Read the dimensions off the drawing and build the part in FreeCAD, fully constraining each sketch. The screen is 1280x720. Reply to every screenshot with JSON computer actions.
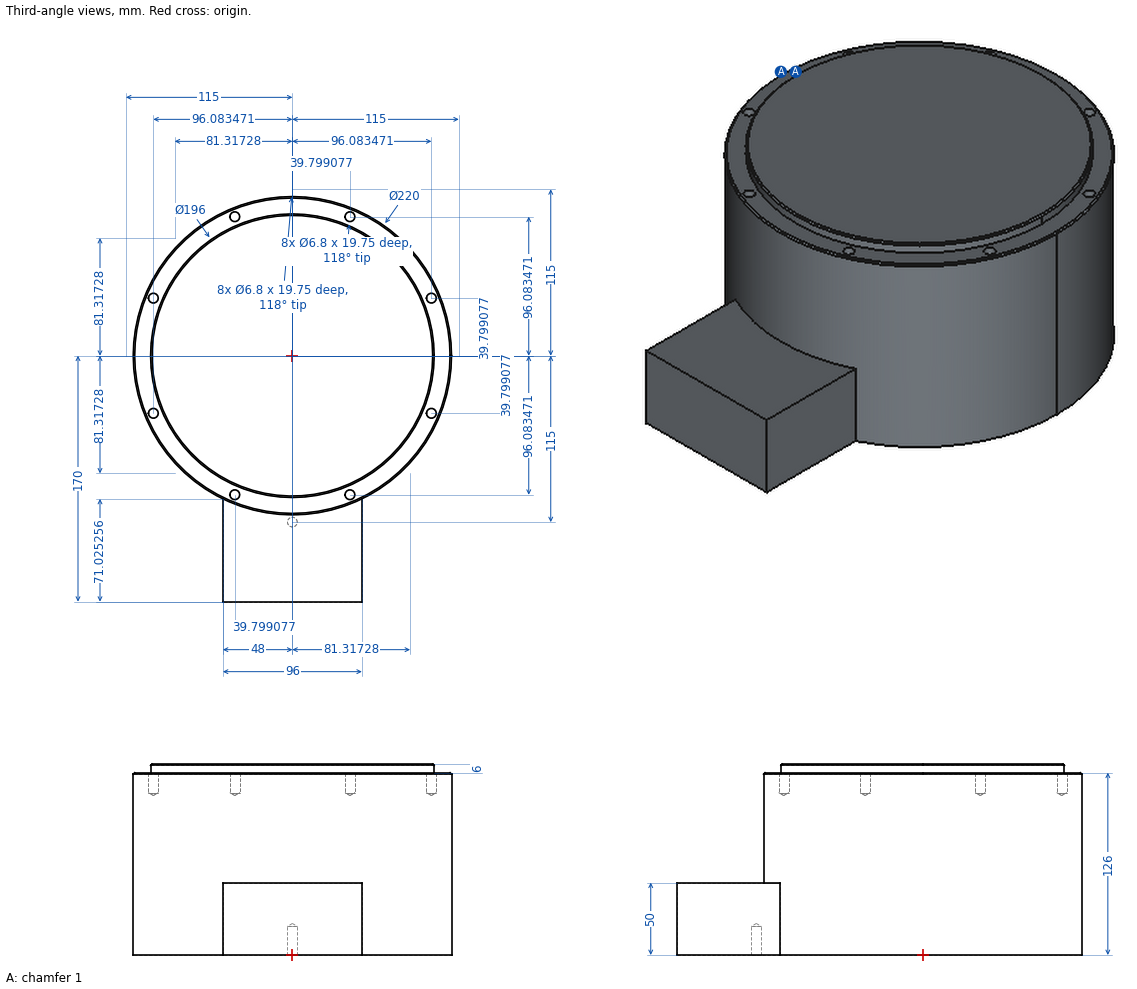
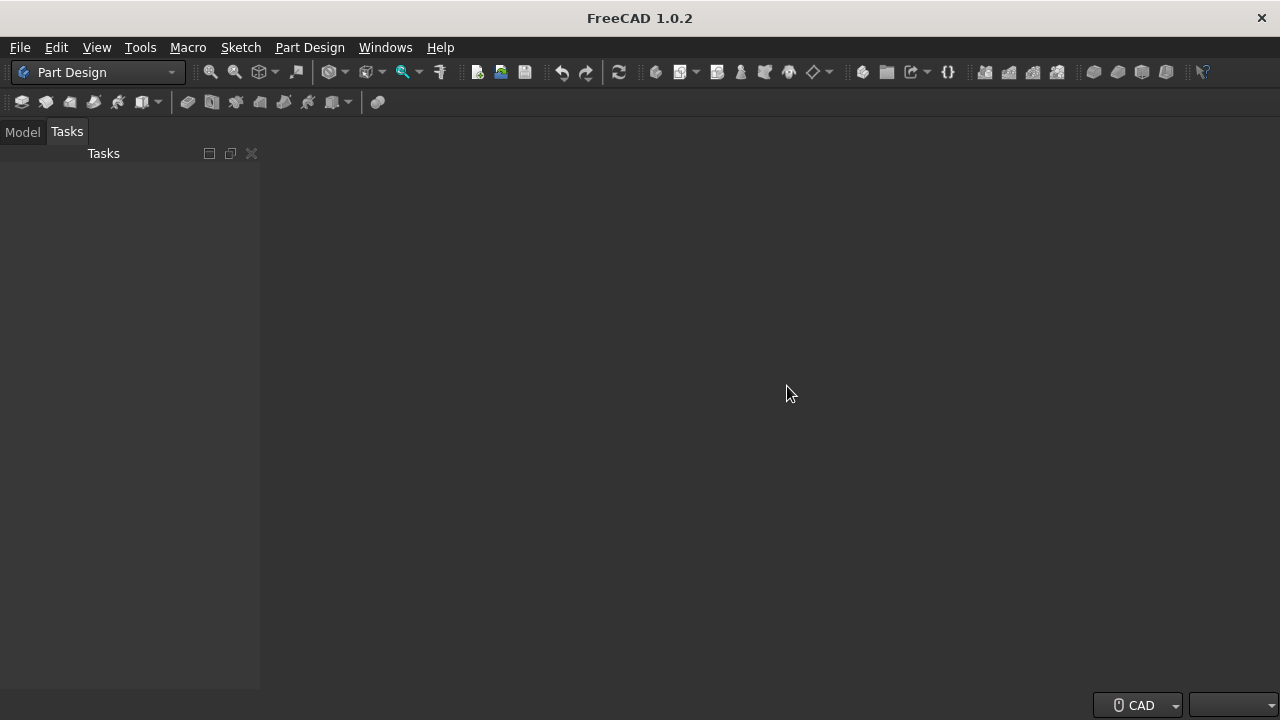
{"action": "left_click", "coordinate": [478, 72]}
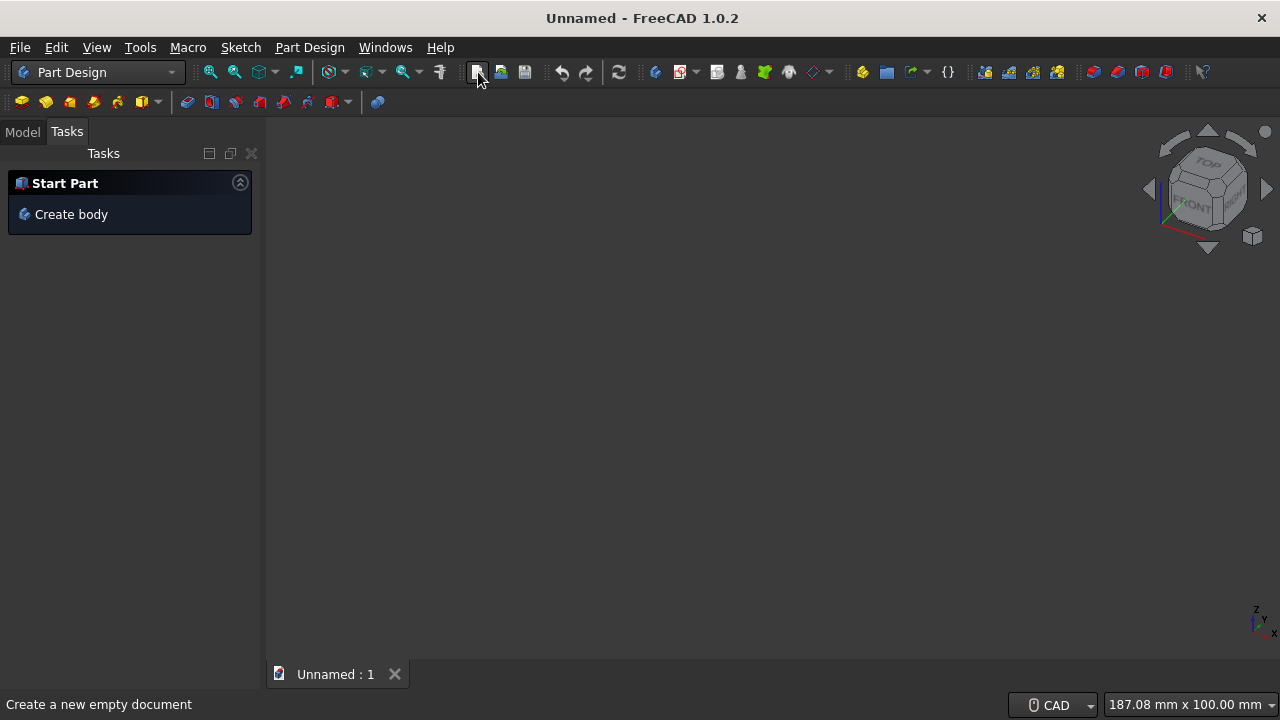
{"action": "left_click", "coordinate": [680, 72]}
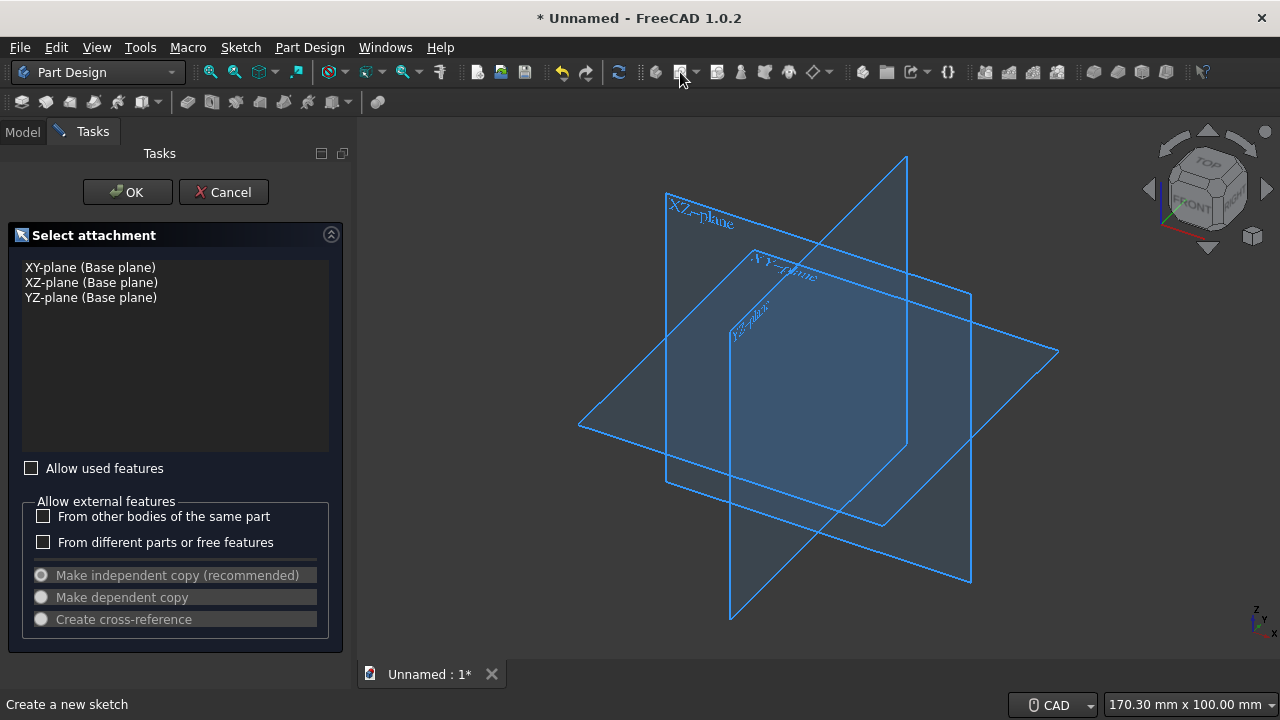
{"action": "left_click", "coordinate": [82, 268]}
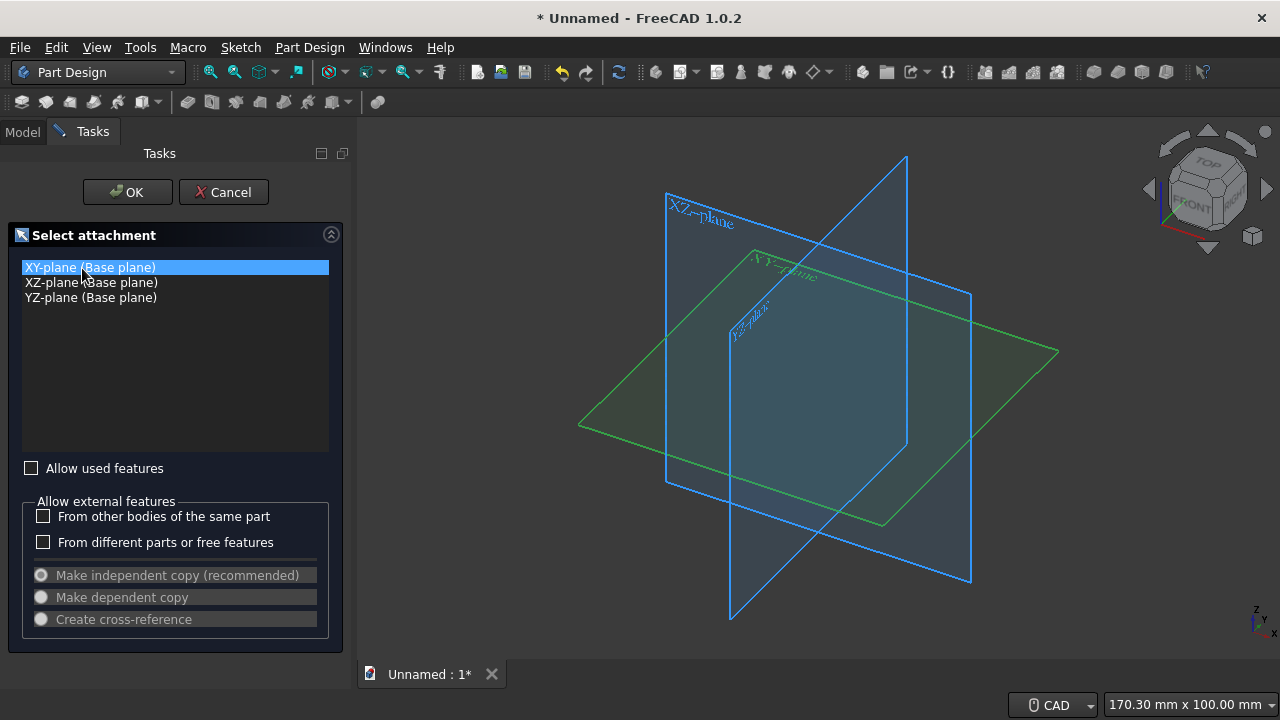
{"action": "left_click", "coordinate": [128, 192]}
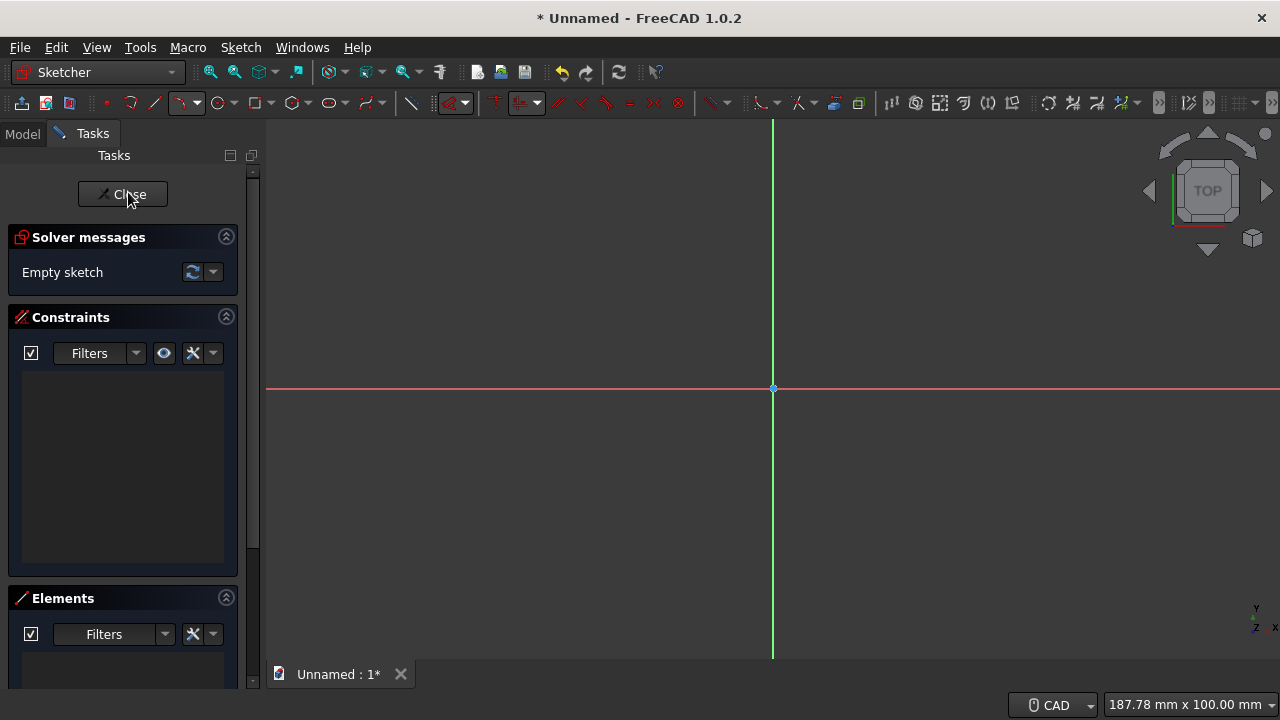
{"action": "scroll", "coordinate": [675, 389], "scroll_direction": "down", "scroll_amount": 6}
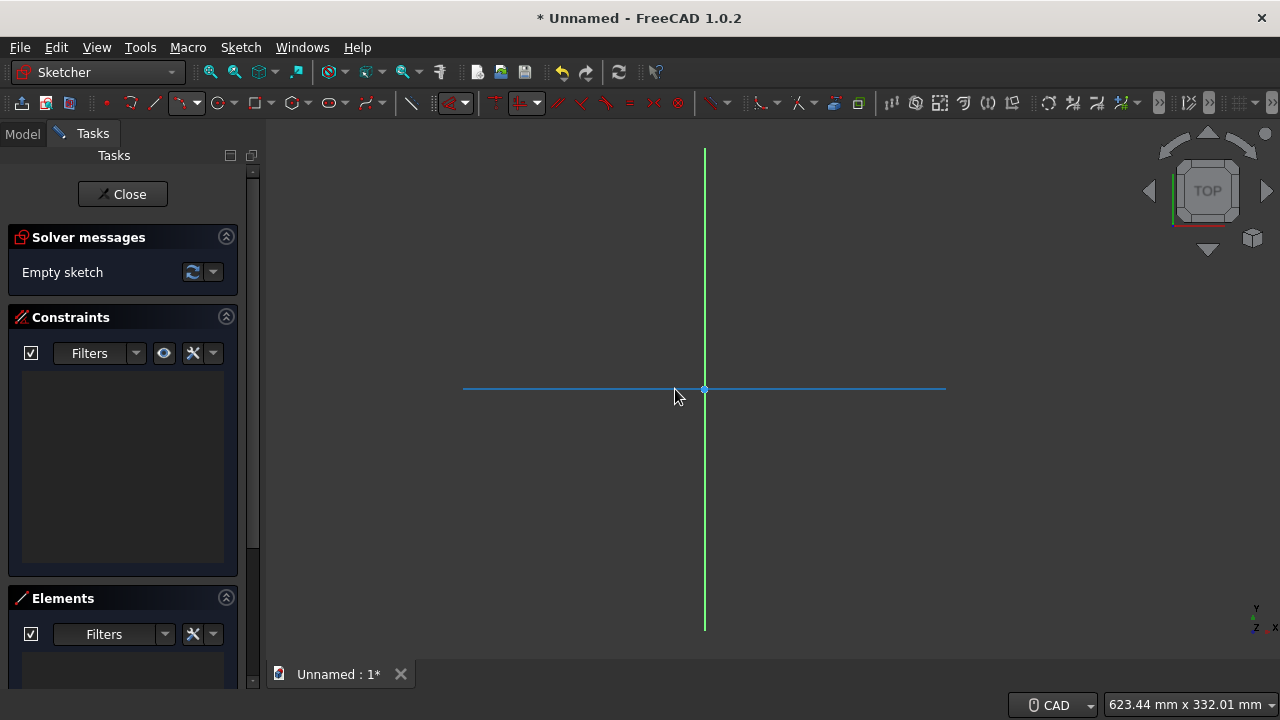
{"action": "left_click", "coordinate": [218, 104]}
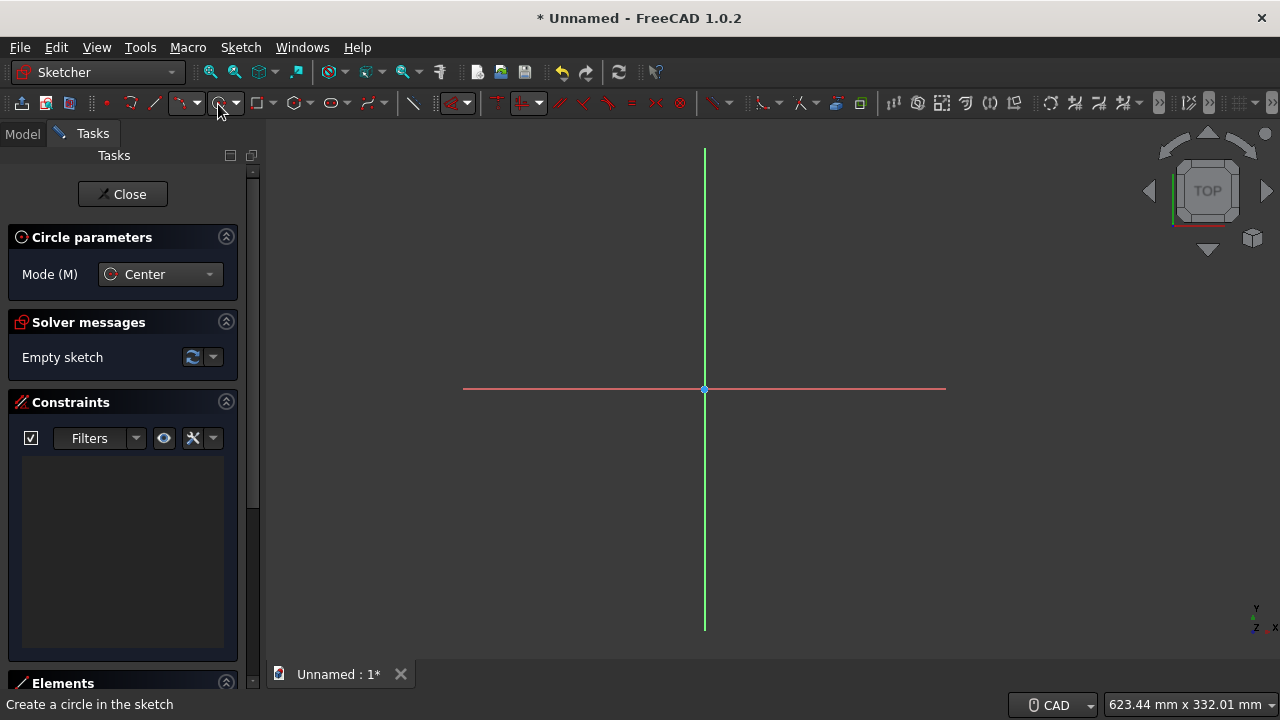
{"action": "left_click", "coordinate": [705, 389]}
{"action": "left_click", "coordinate": [831, 263]}
{"action": "key", "text": "Escape"}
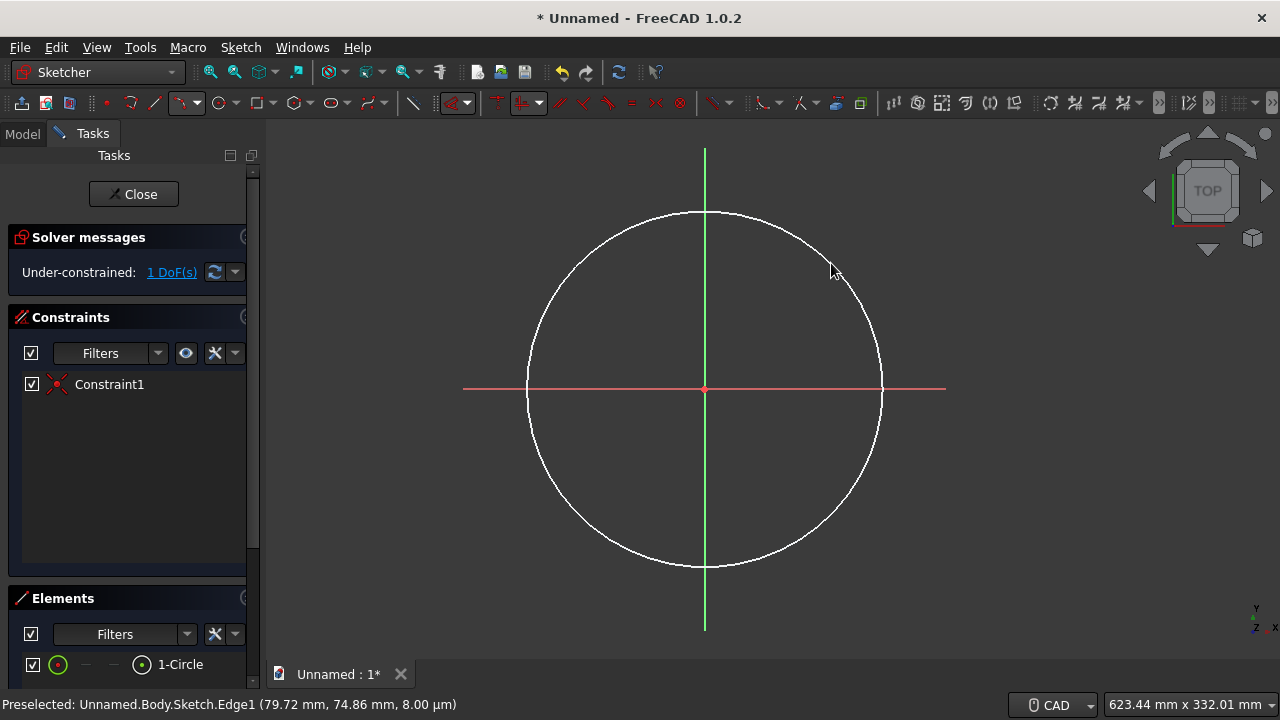
{"action": "left_click", "coordinate": [452, 104]}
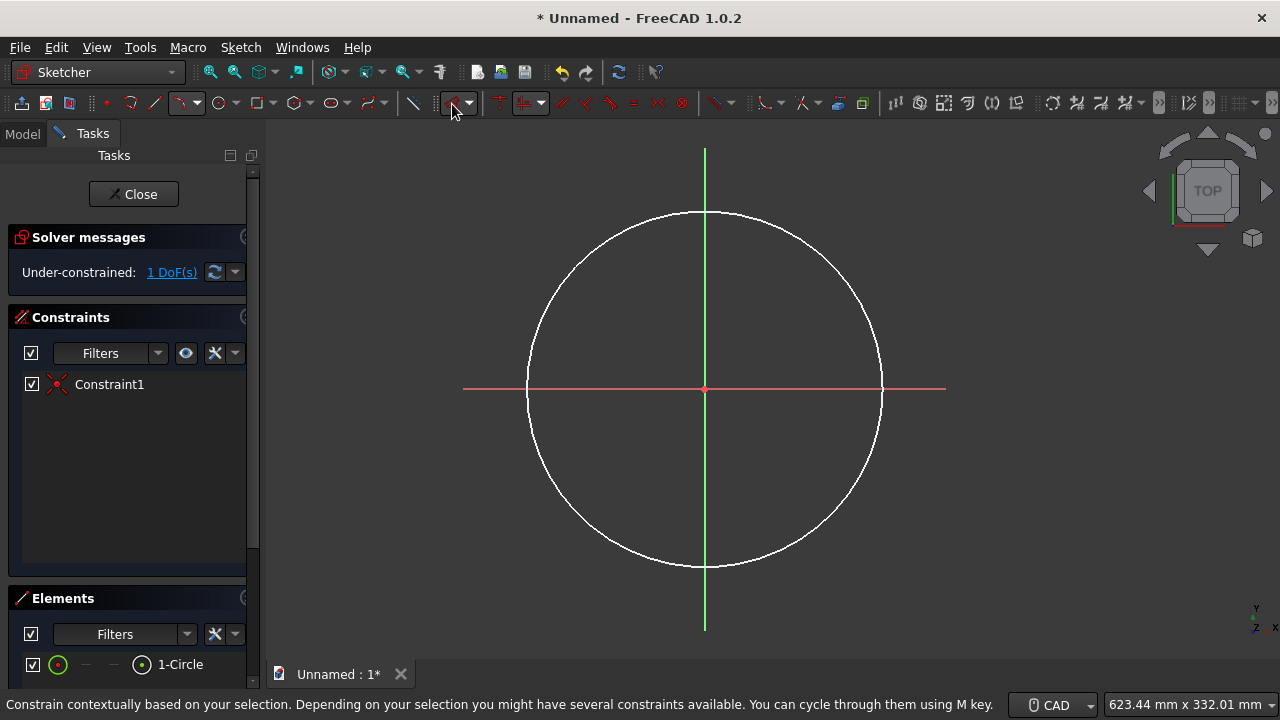
{"action": "left_click", "coordinate": [830, 263]}
{"action": "left_click", "coordinate": [853, 240]}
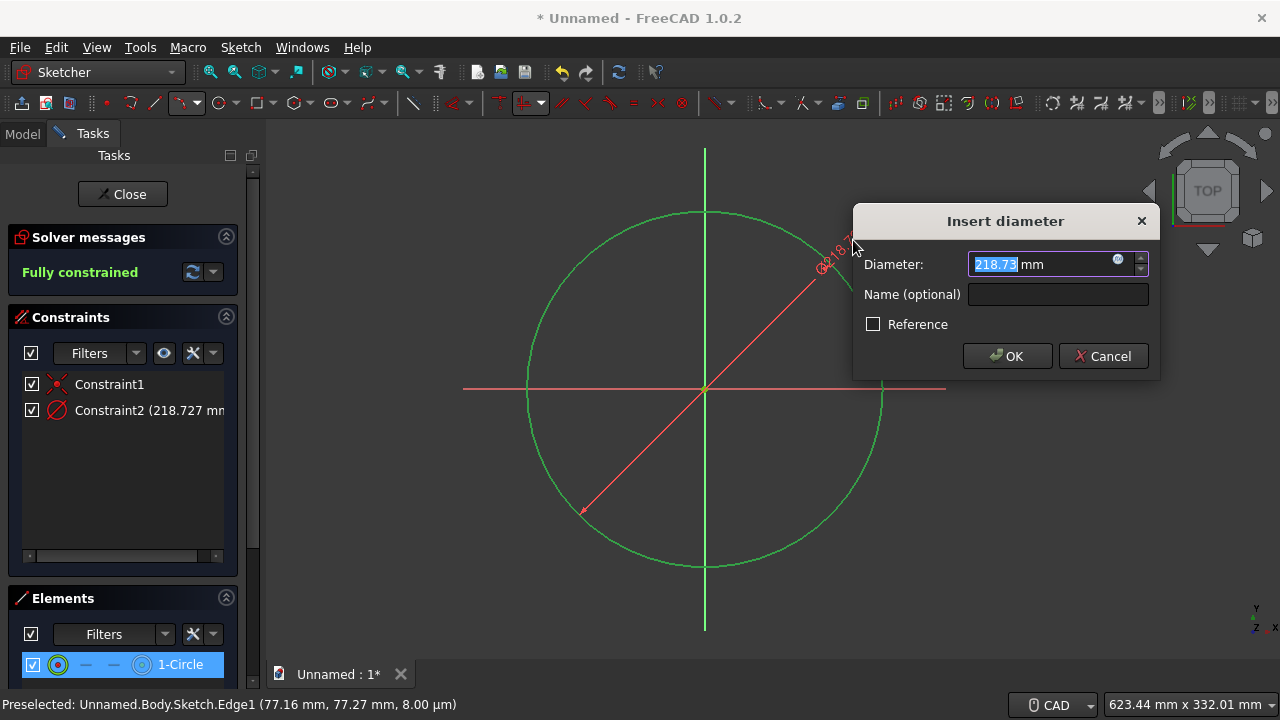
{"action": "type", "text": "220"}
{"action": "key", "text": "Return"}
{"action": "key", "text": "Escape"}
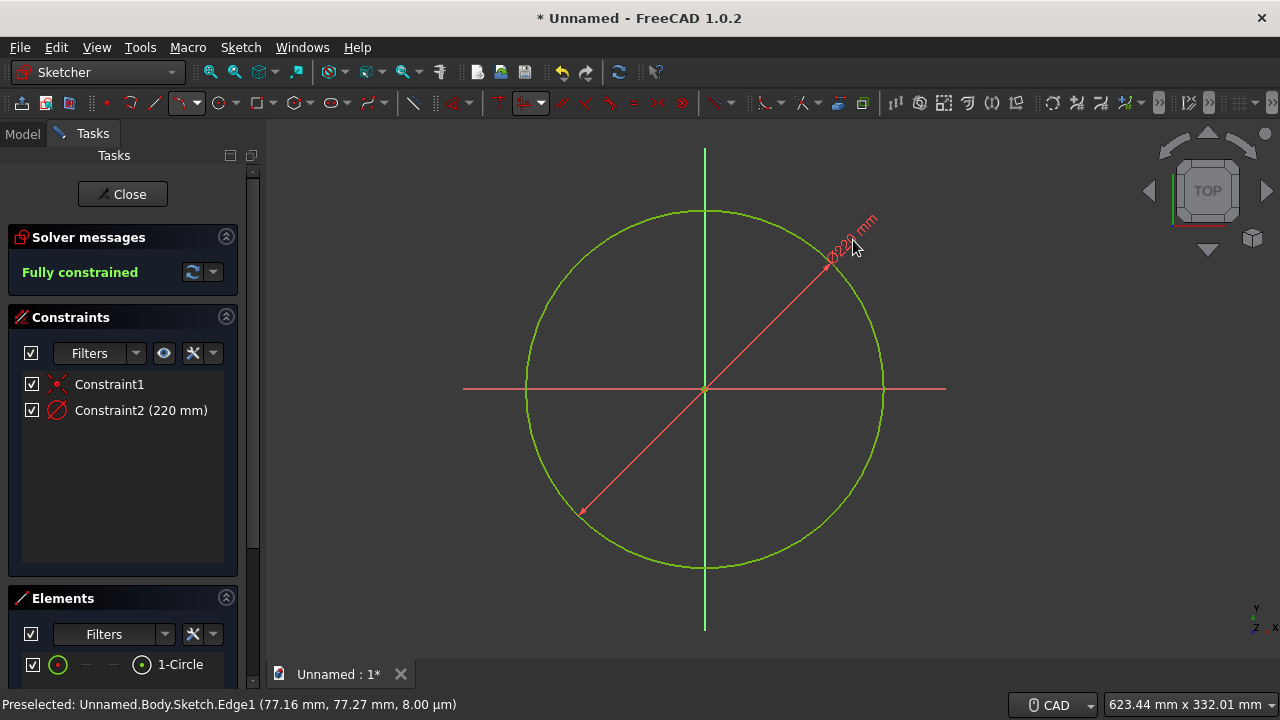
{"action": "left_click", "coordinate": [123, 194]}